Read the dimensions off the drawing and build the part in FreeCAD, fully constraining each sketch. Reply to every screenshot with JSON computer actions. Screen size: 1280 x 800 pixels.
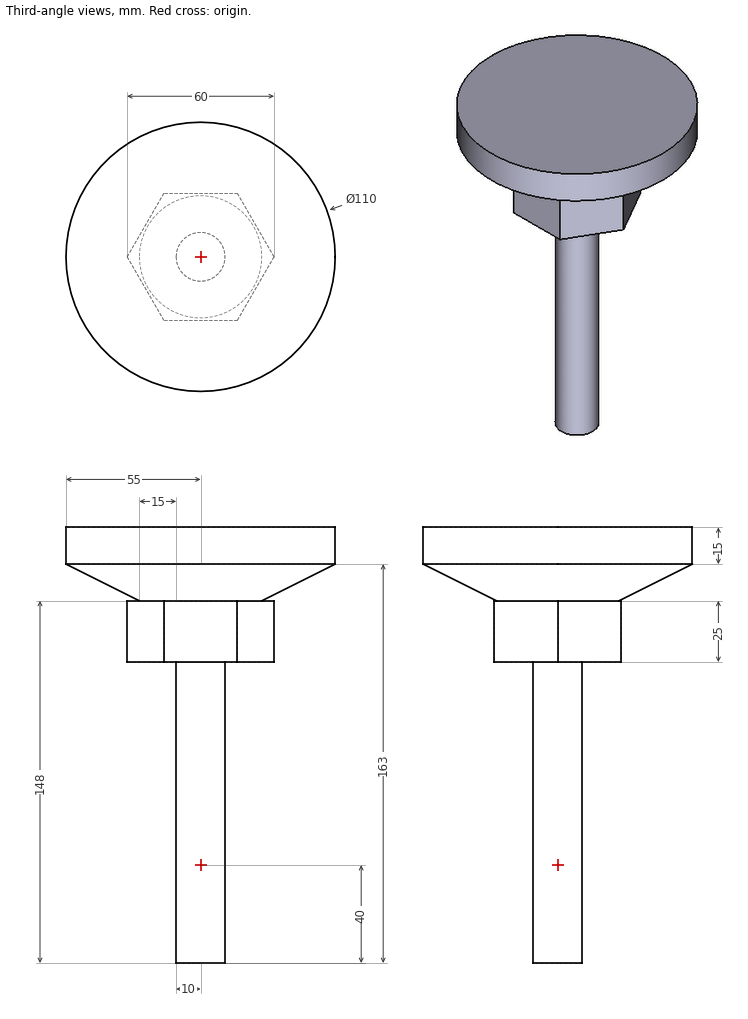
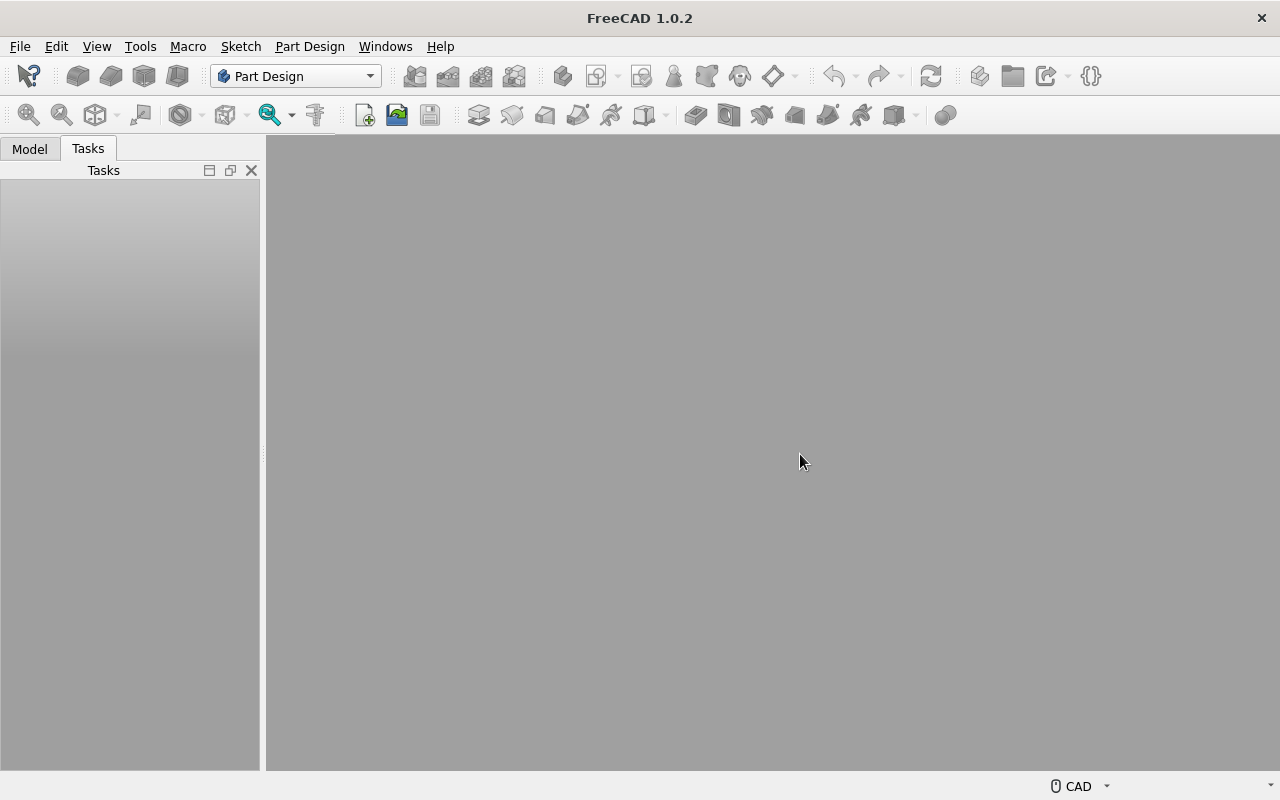
{"action": "left_click", "coordinate": [364, 116]}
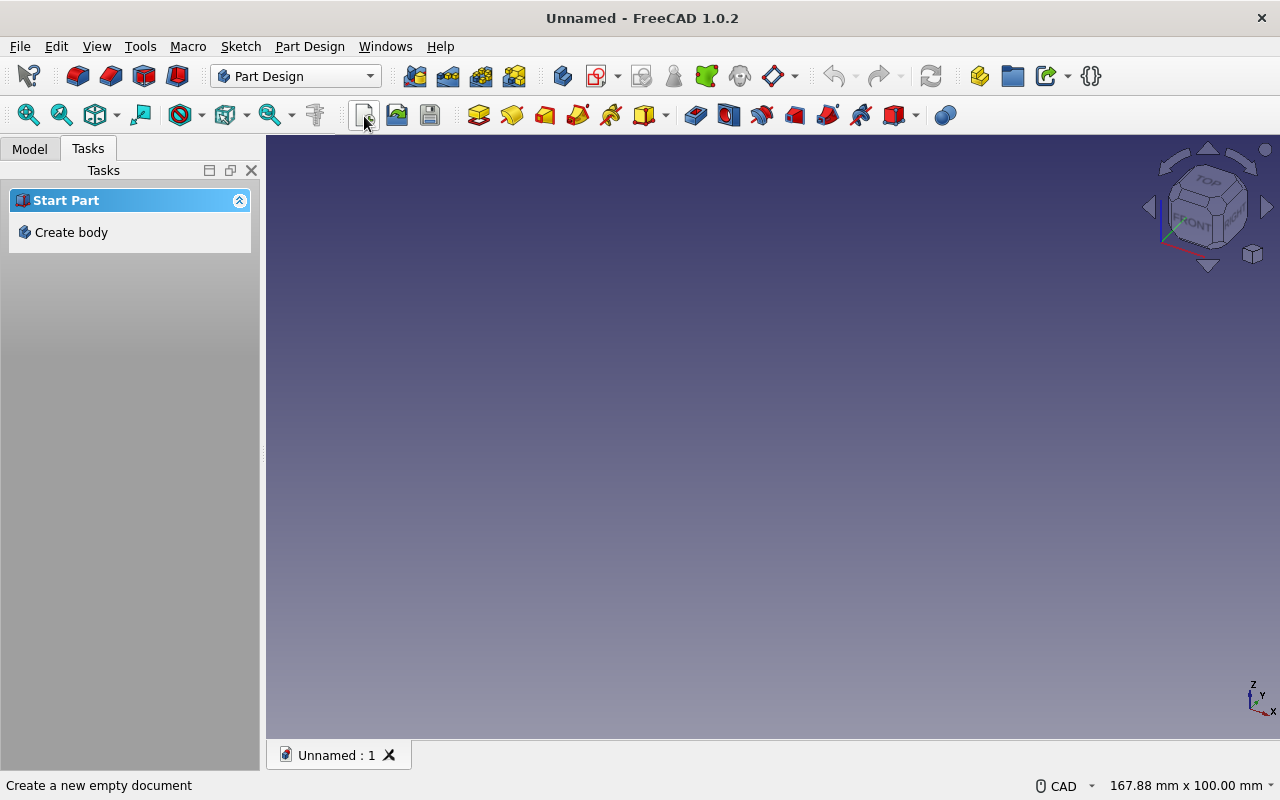
{"action": "left_click", "coordinate": [596, 76]}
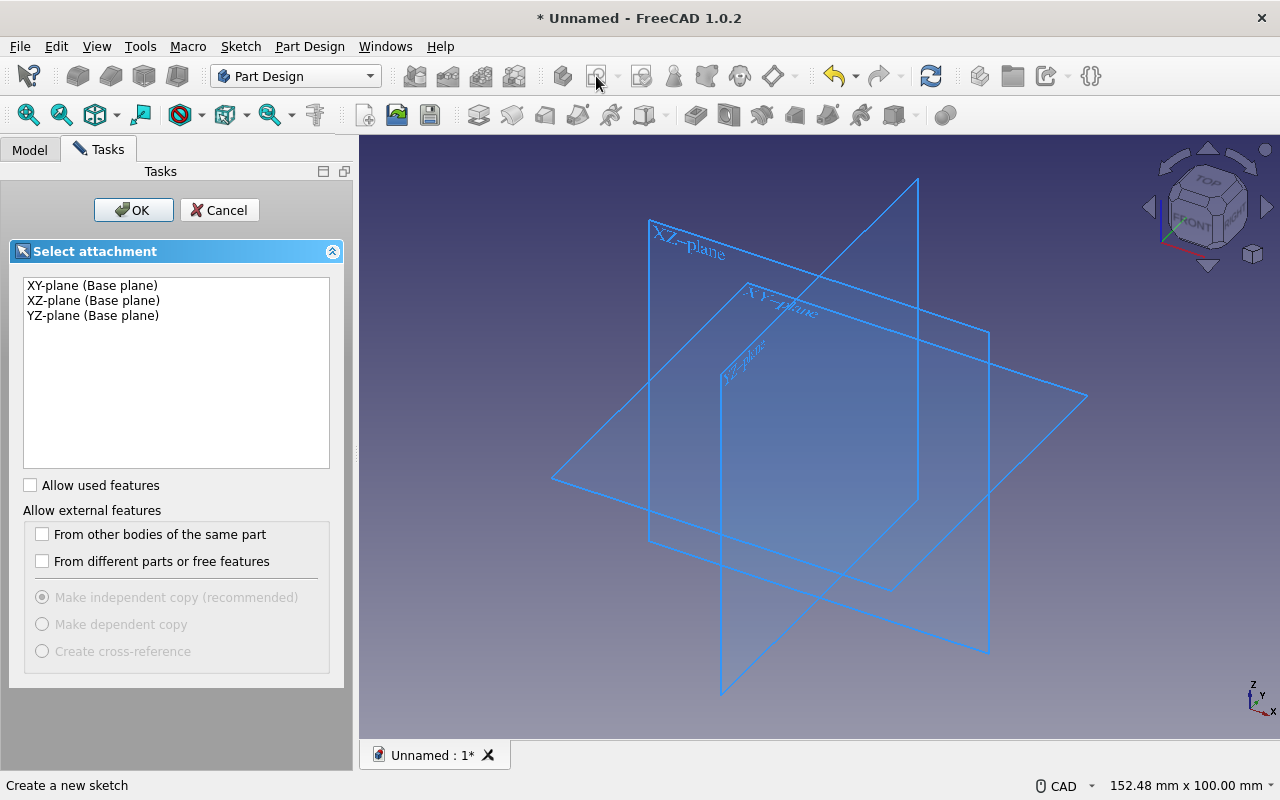
{"action": "left_click", "coordinate": [84, 300]}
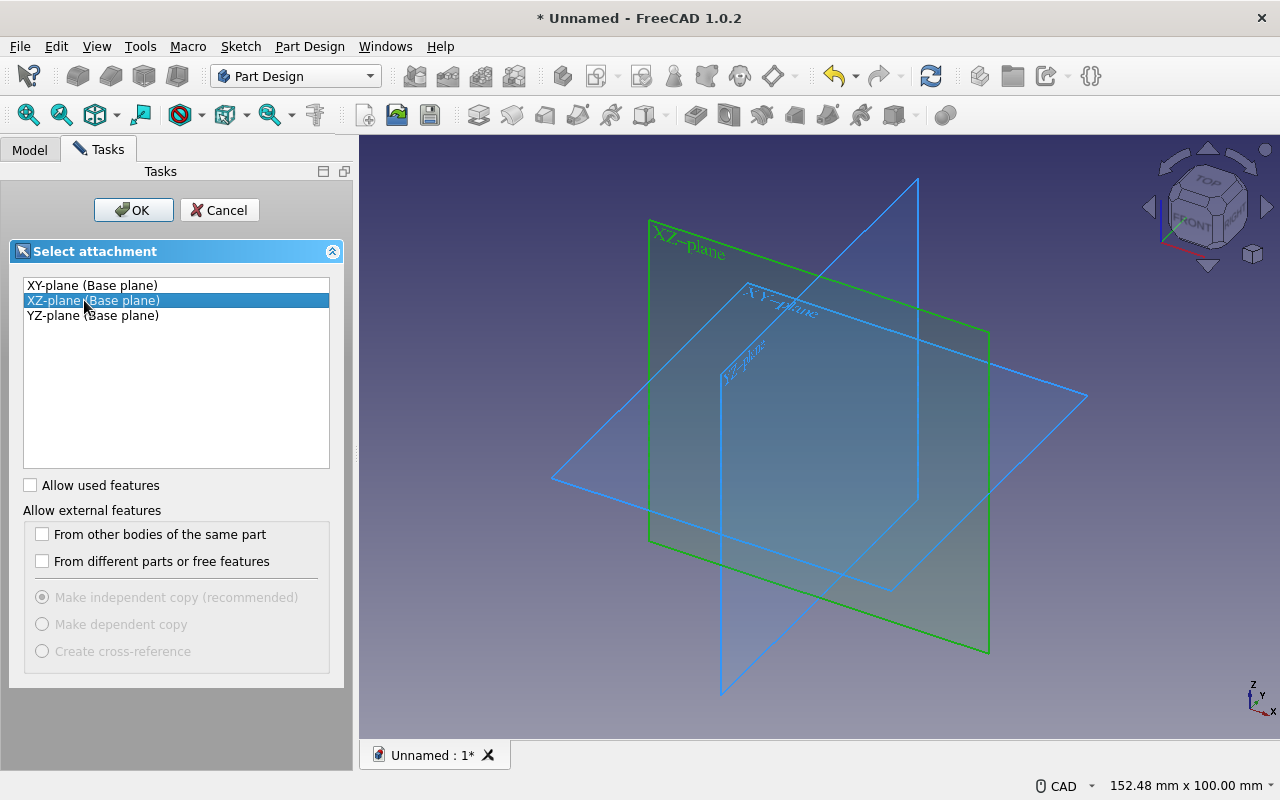
{"action": "left_click", "coordinate": [134, 210]}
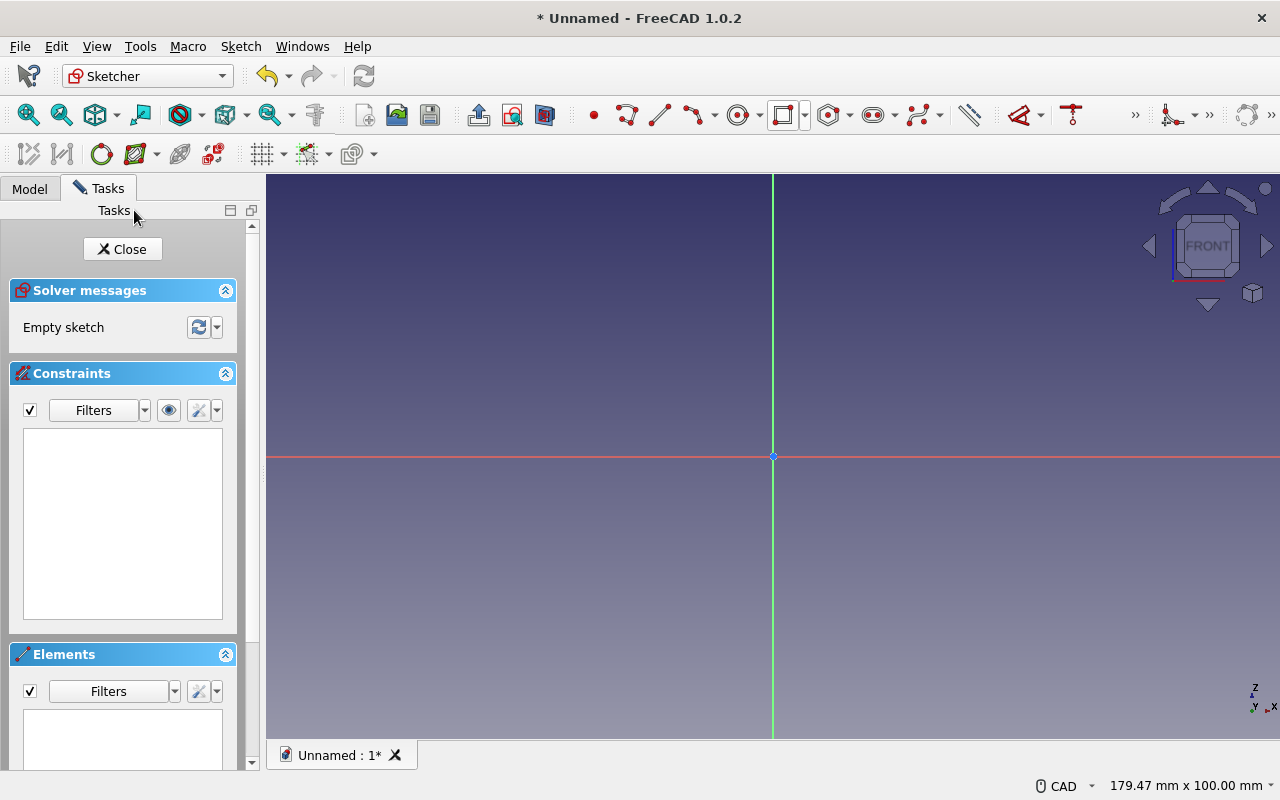
{"action": "scroll", "coordinate": [755, 593], "scroll_direction": "down", "scroll_amount": 5}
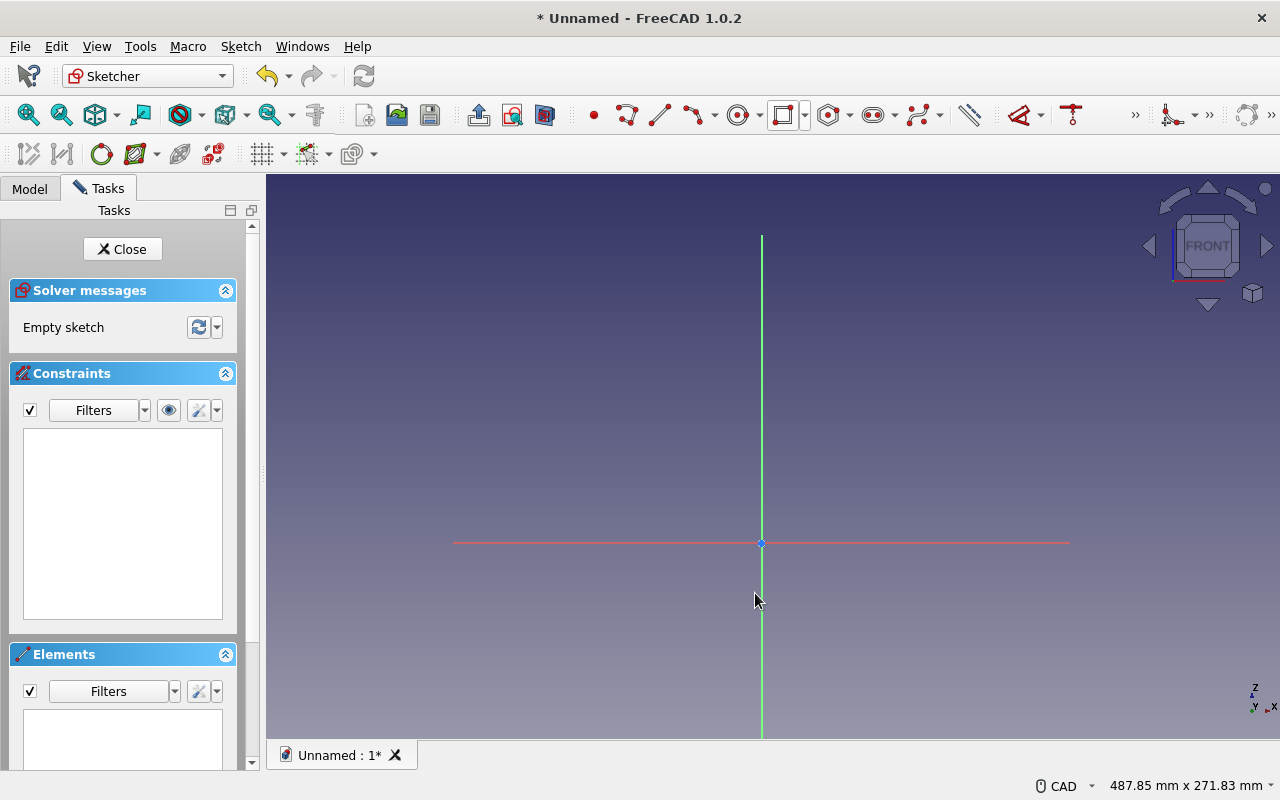
{"action": "left_click", "coordinate": [627, 116]}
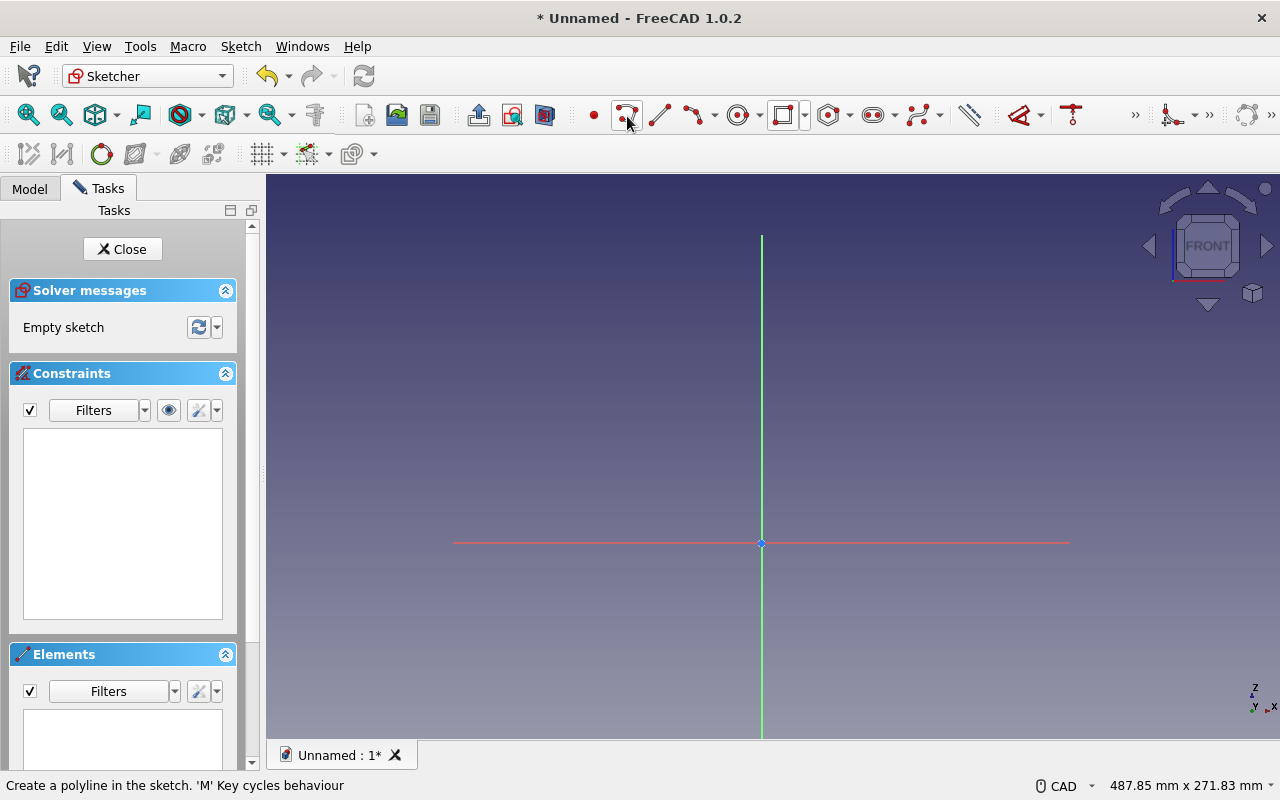
{"action": "left_click", "coordinate": [762, 626]}
{"action": "left_click", "coordinate": [741, 626]}
{"action": "left_click", "coordinate": [741, 319]}
{"action": "left_click", "coordinate": [710, 319]}
{"action": "left_click", "coordinate": [648, 288]}
{"action": "left_click", "coordinate": [753, 288]}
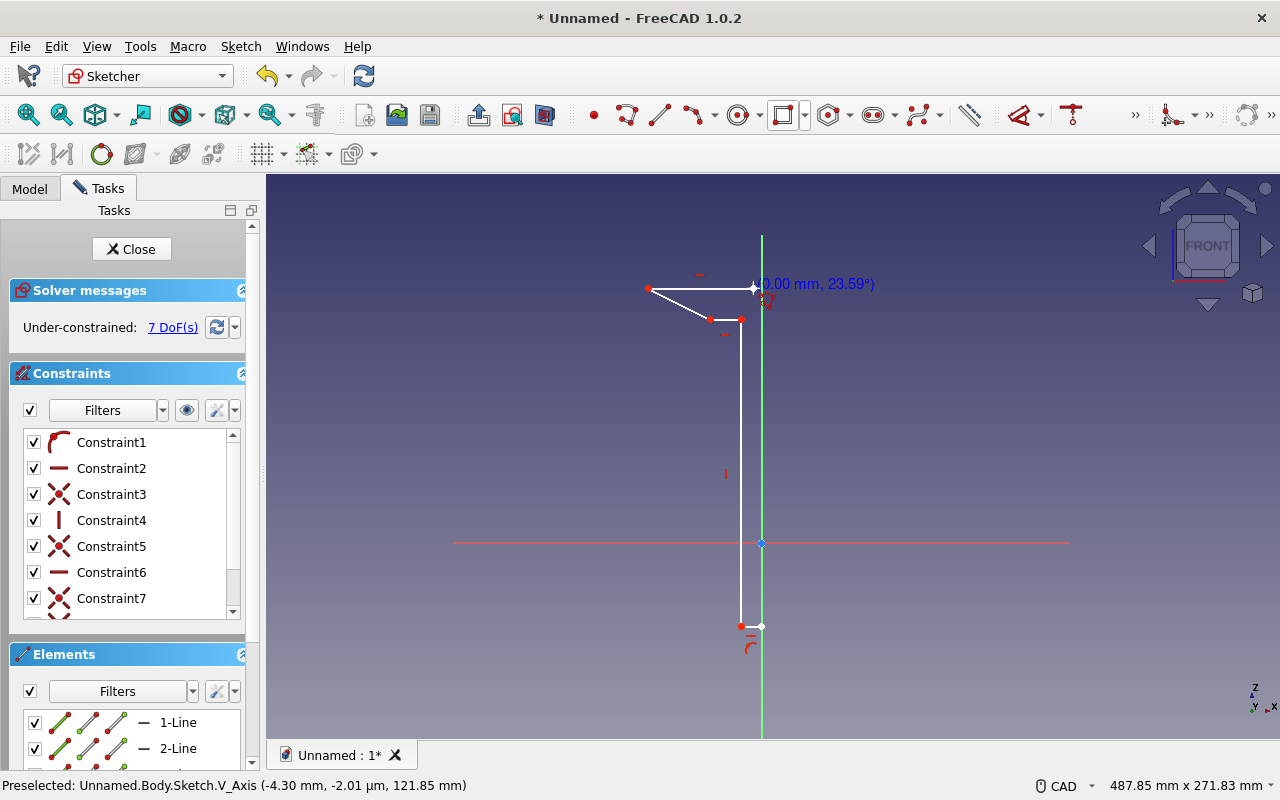
{"action": "scroll", "coordinate": [762, 626], "scroll_direction": "up", "scroll_amount": 3}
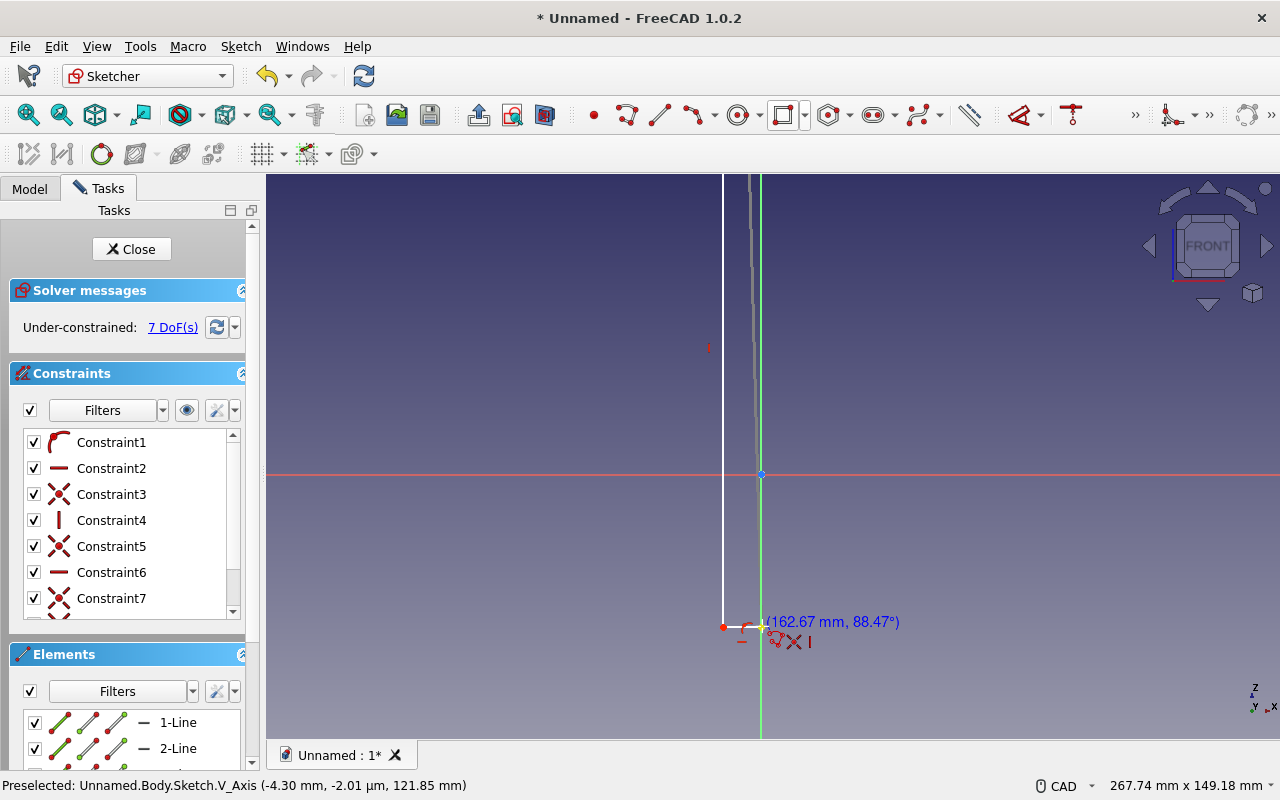
{"action": "left_click", "coordinate": [761, 627]}
{"action": "key", "text": "Escape"}
{"action": "key", "text": "Escape"}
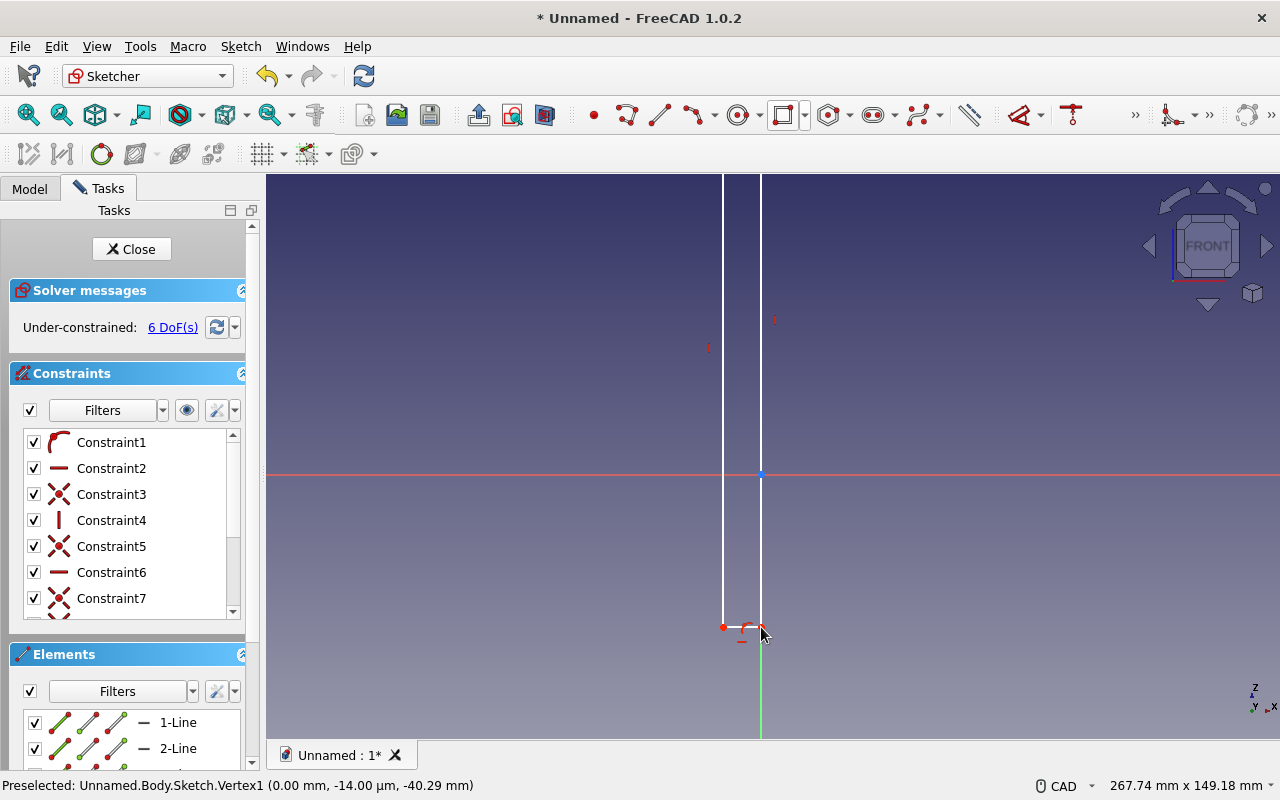
{"action": "left_click", "coordinate": [735, 627]}